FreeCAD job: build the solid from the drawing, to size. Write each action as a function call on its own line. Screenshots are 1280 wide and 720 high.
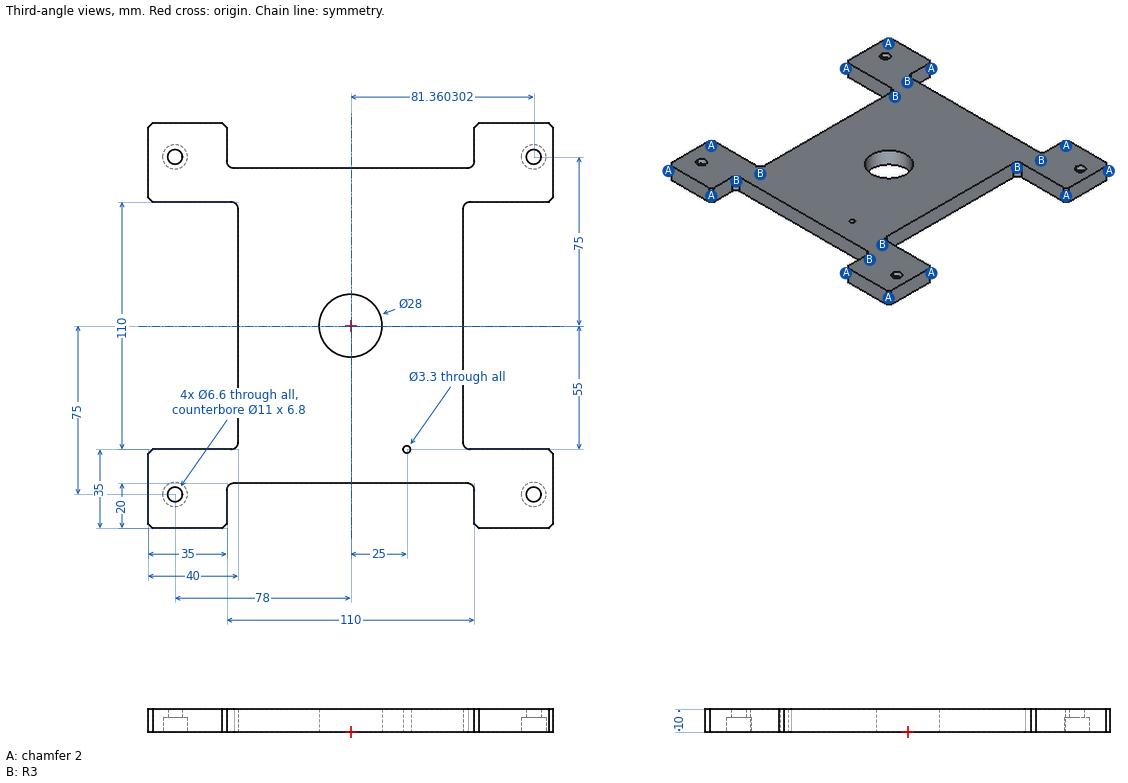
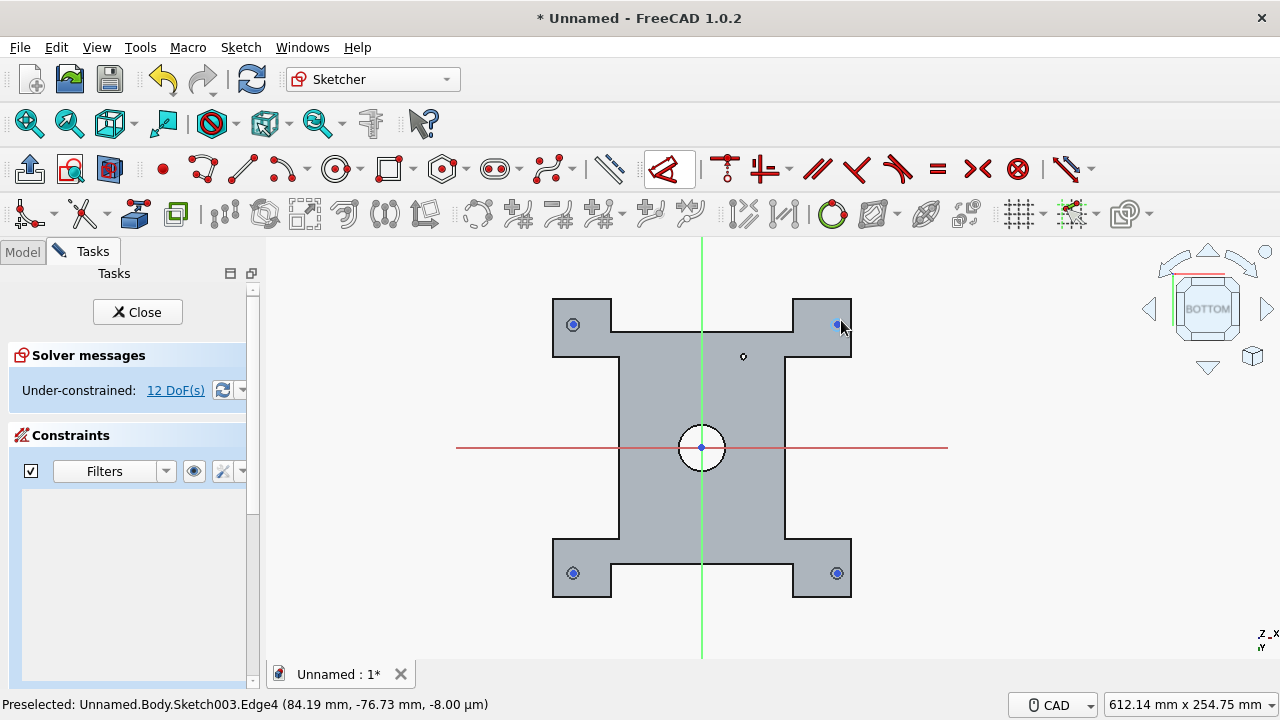
scroll(577, 321, up, 5)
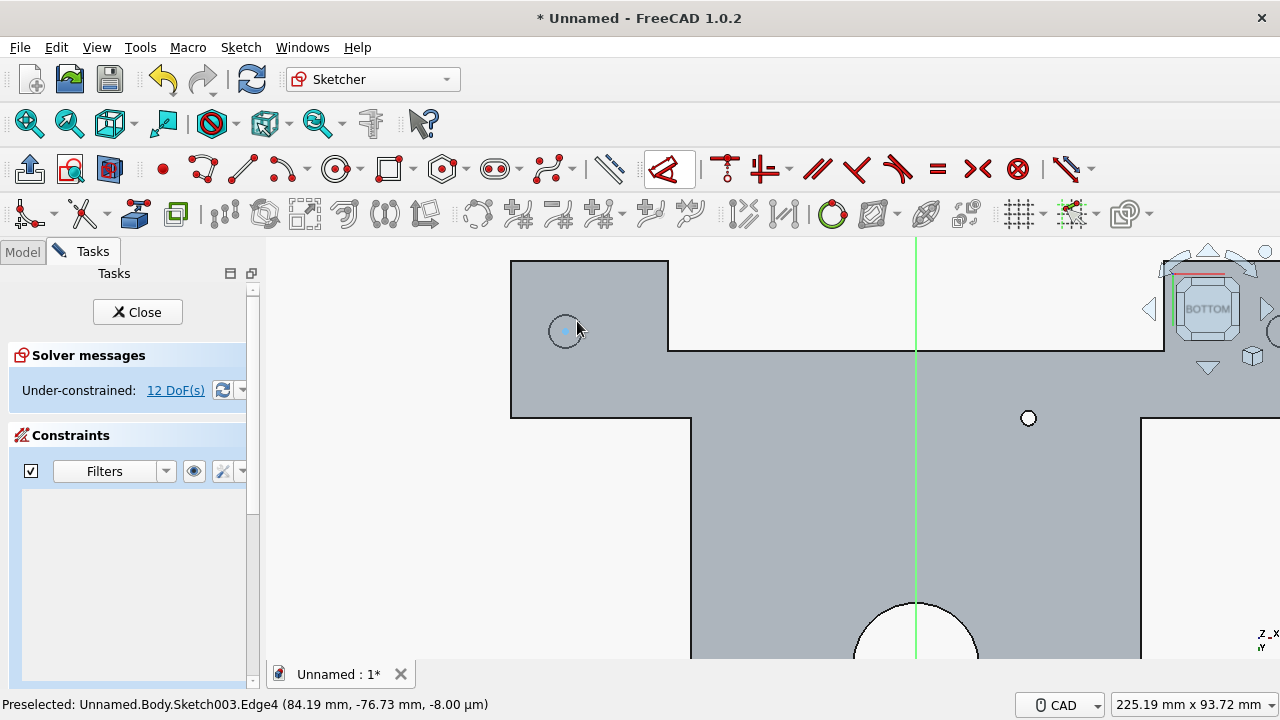
click(577, 320)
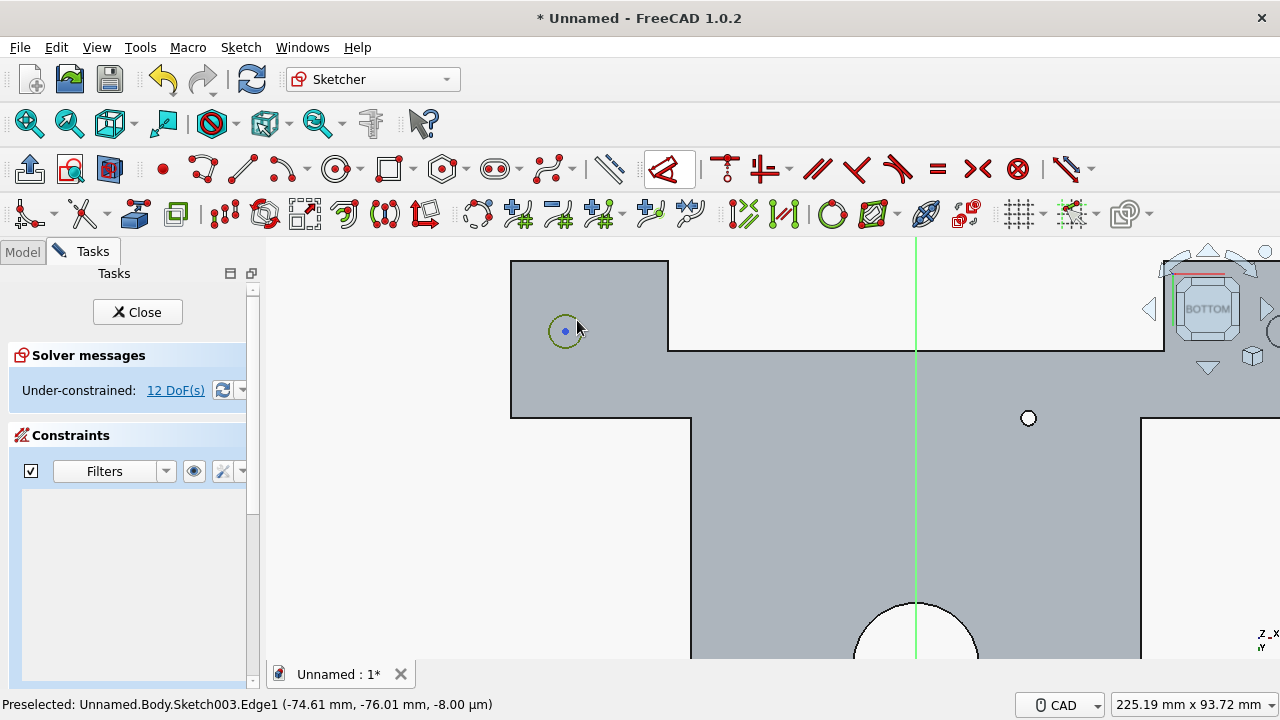
scroll(577, 321, down, 5)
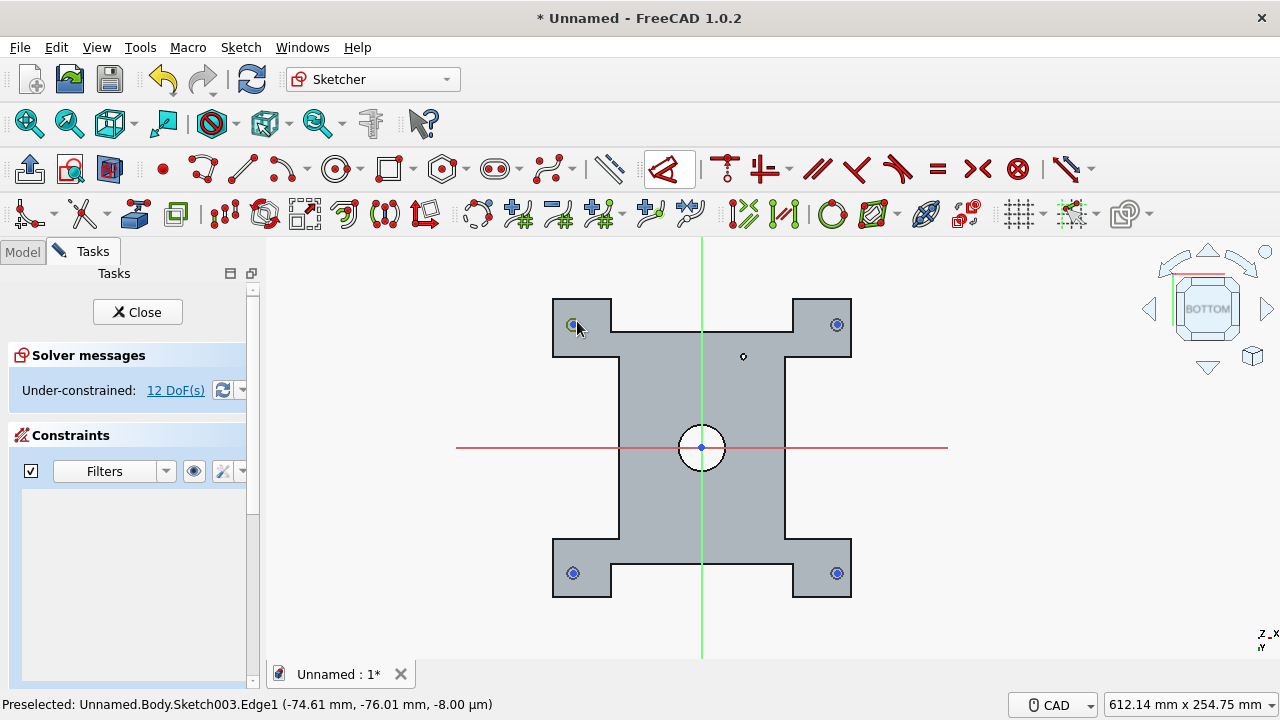
scroll(577, 569, up, 5)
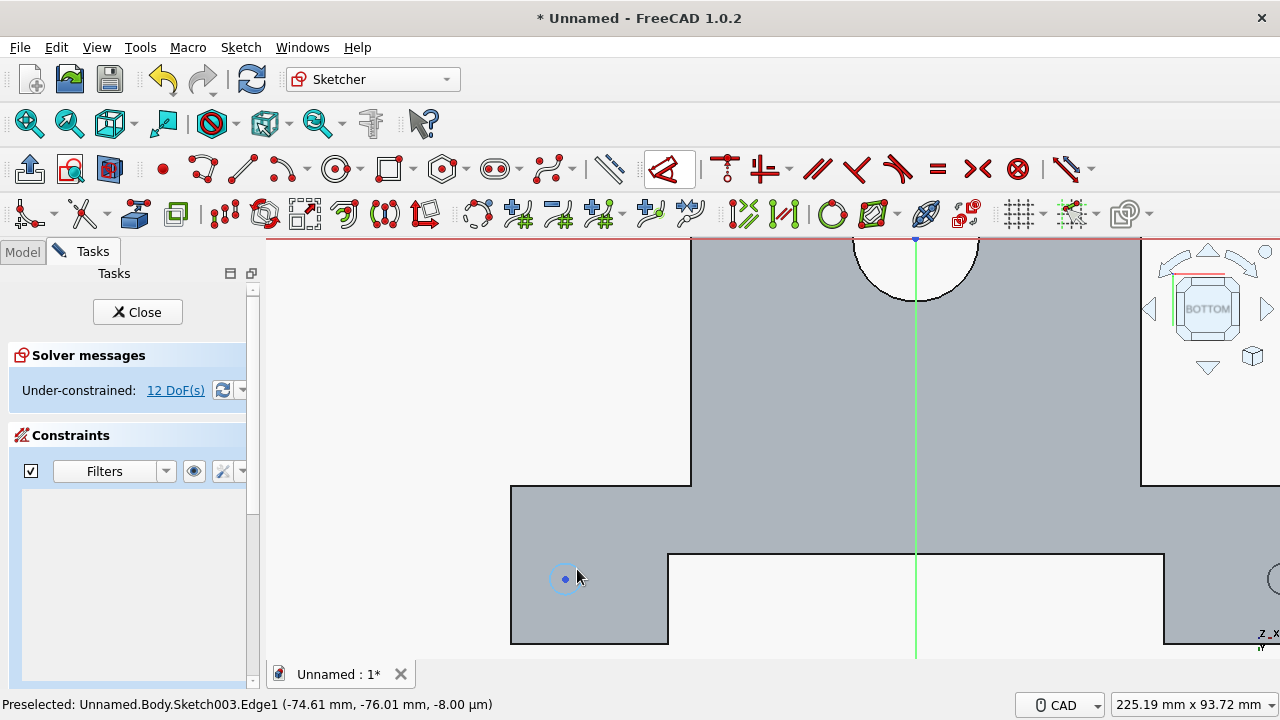
click(577, 568)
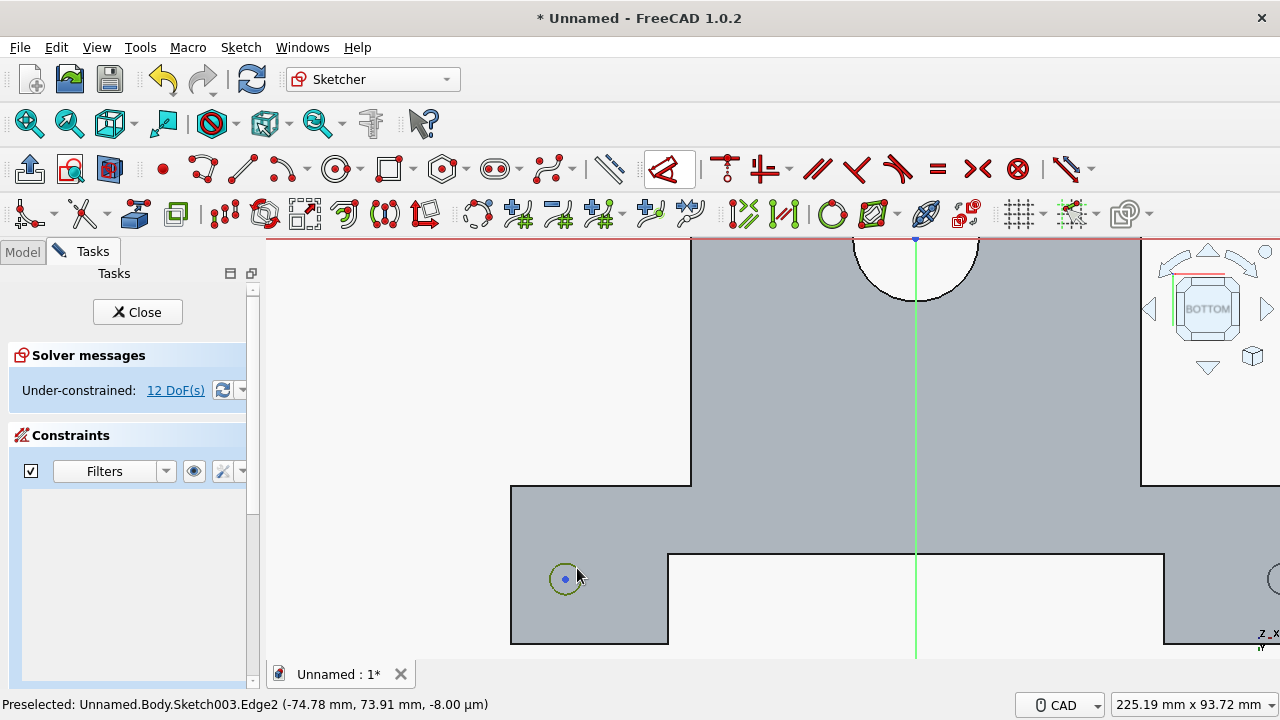
scroll(577, 570, down, 5)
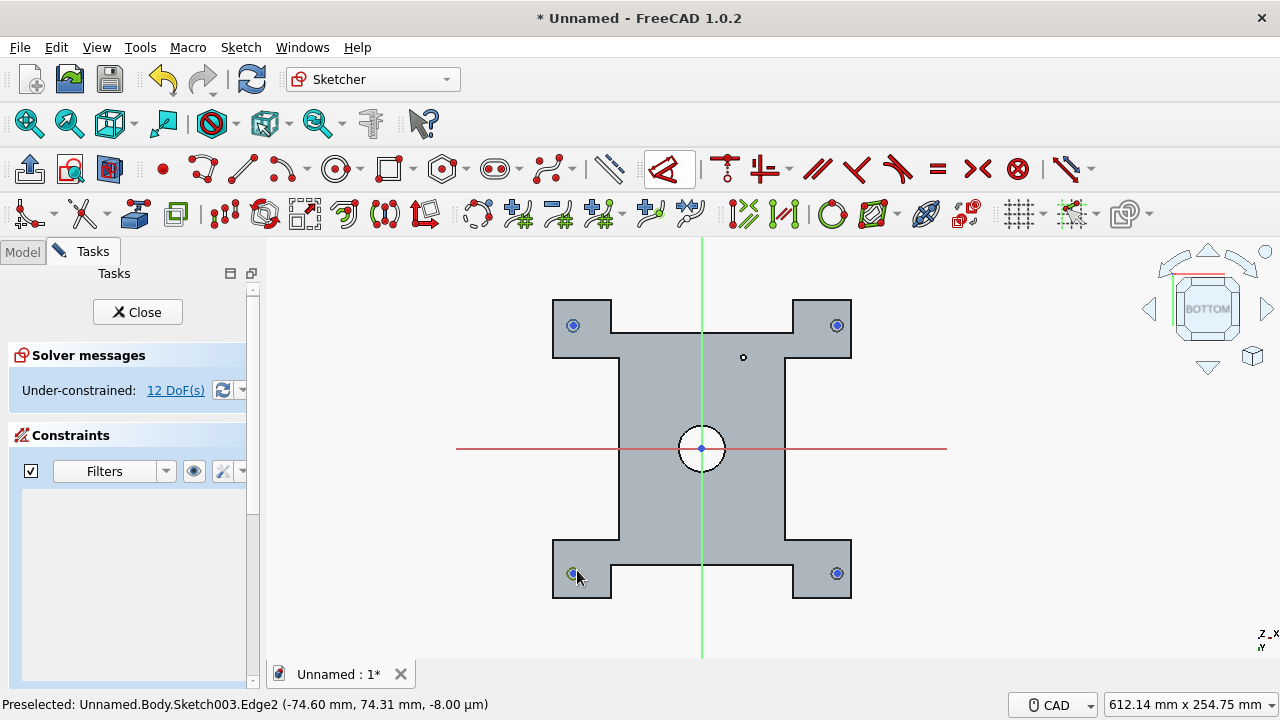
scroll(841, 570, up, 5)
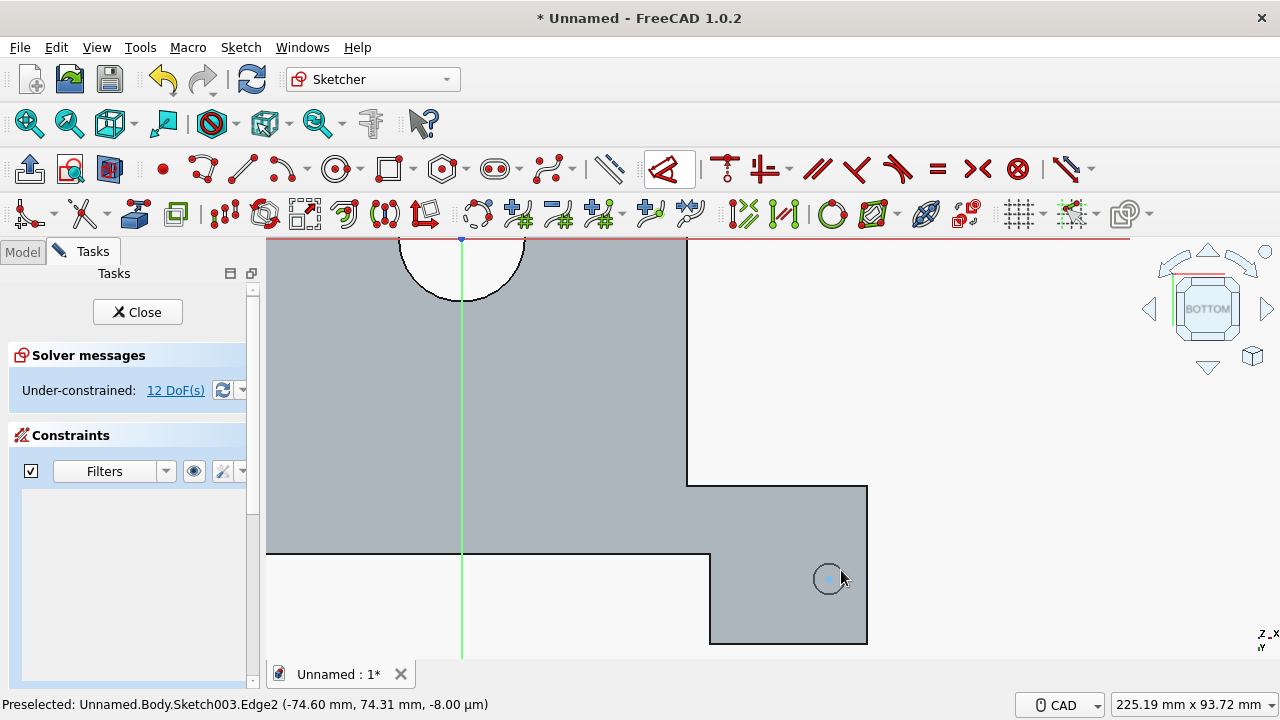
click(840, 568)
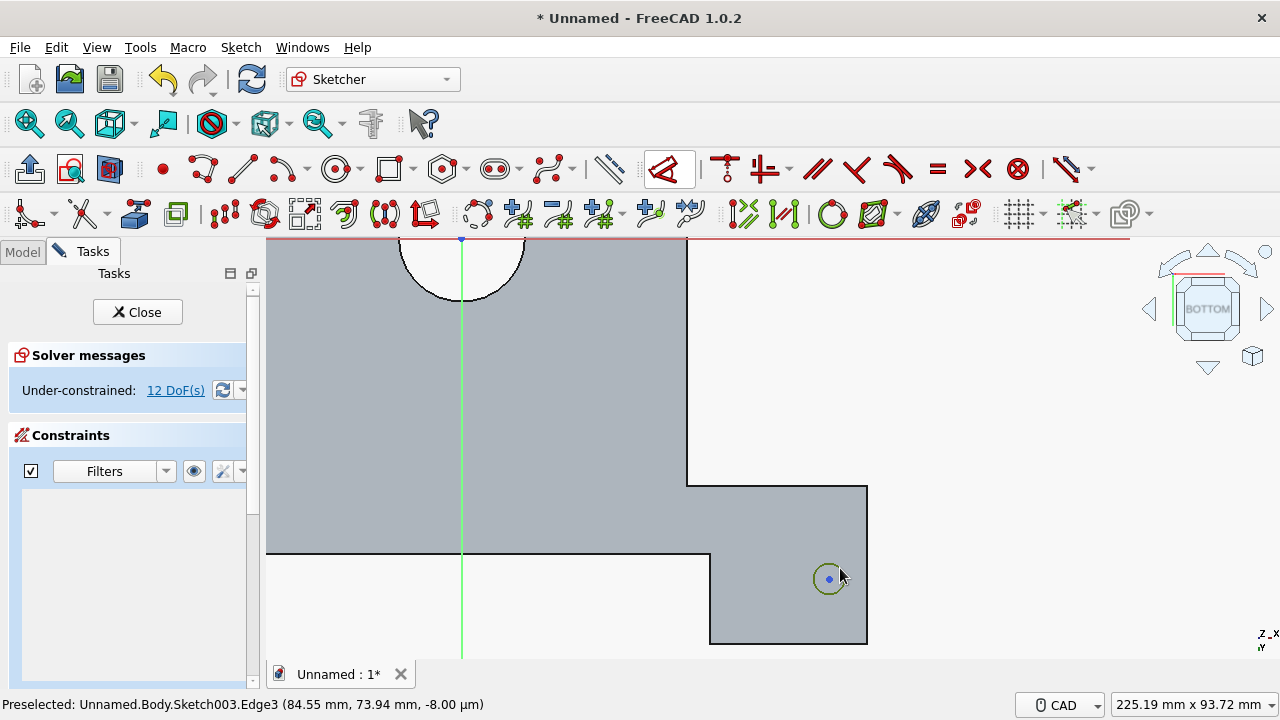
scroll(841, 570, down, 5)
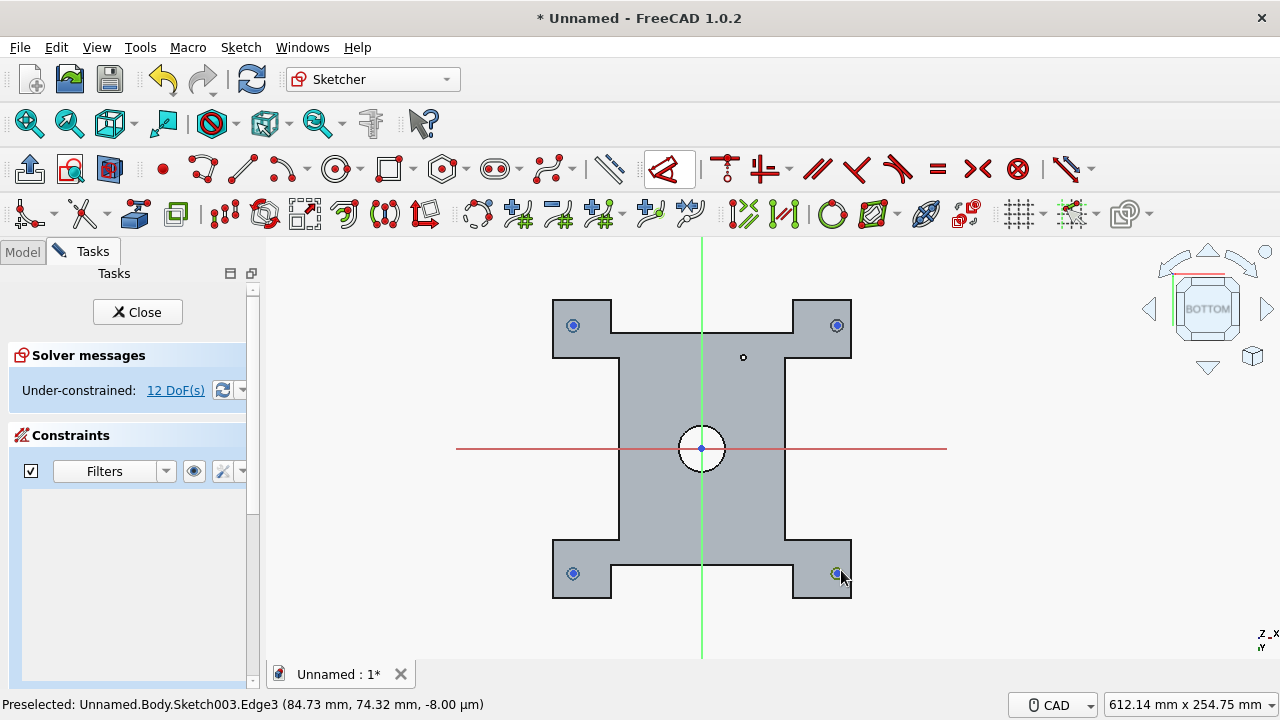
scroll(841, 321, up, 5)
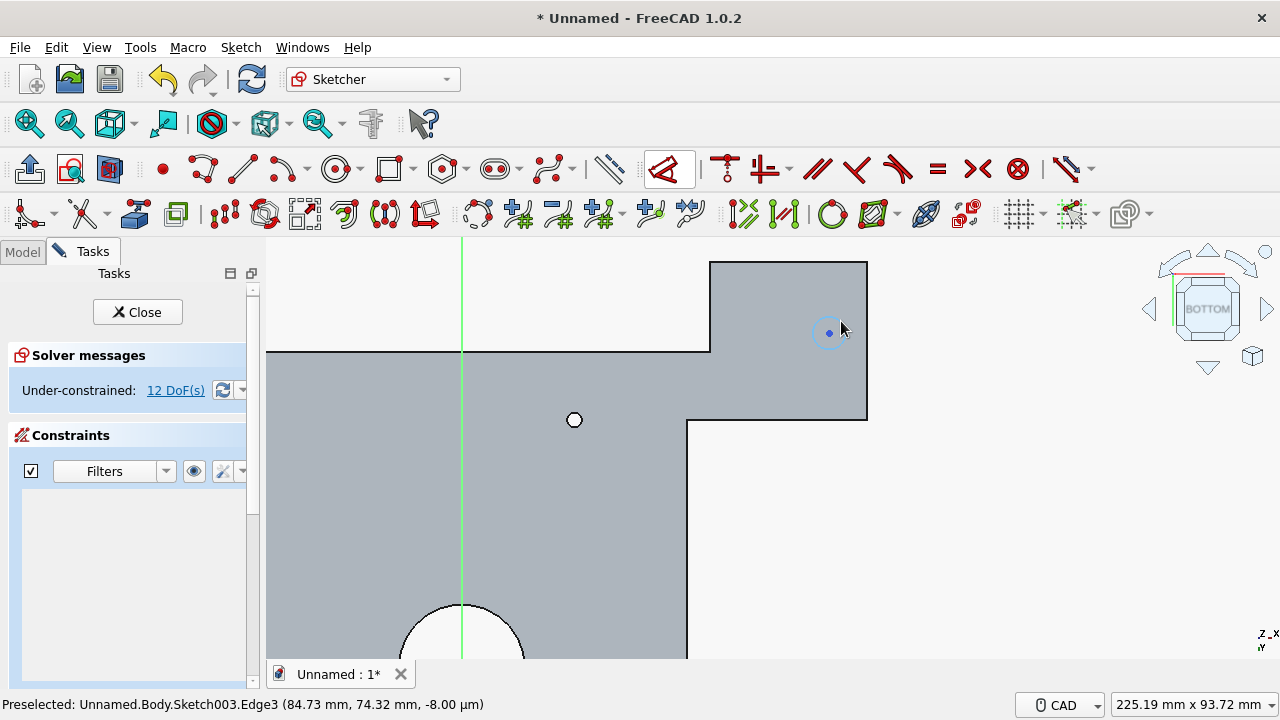
click(841, 322)